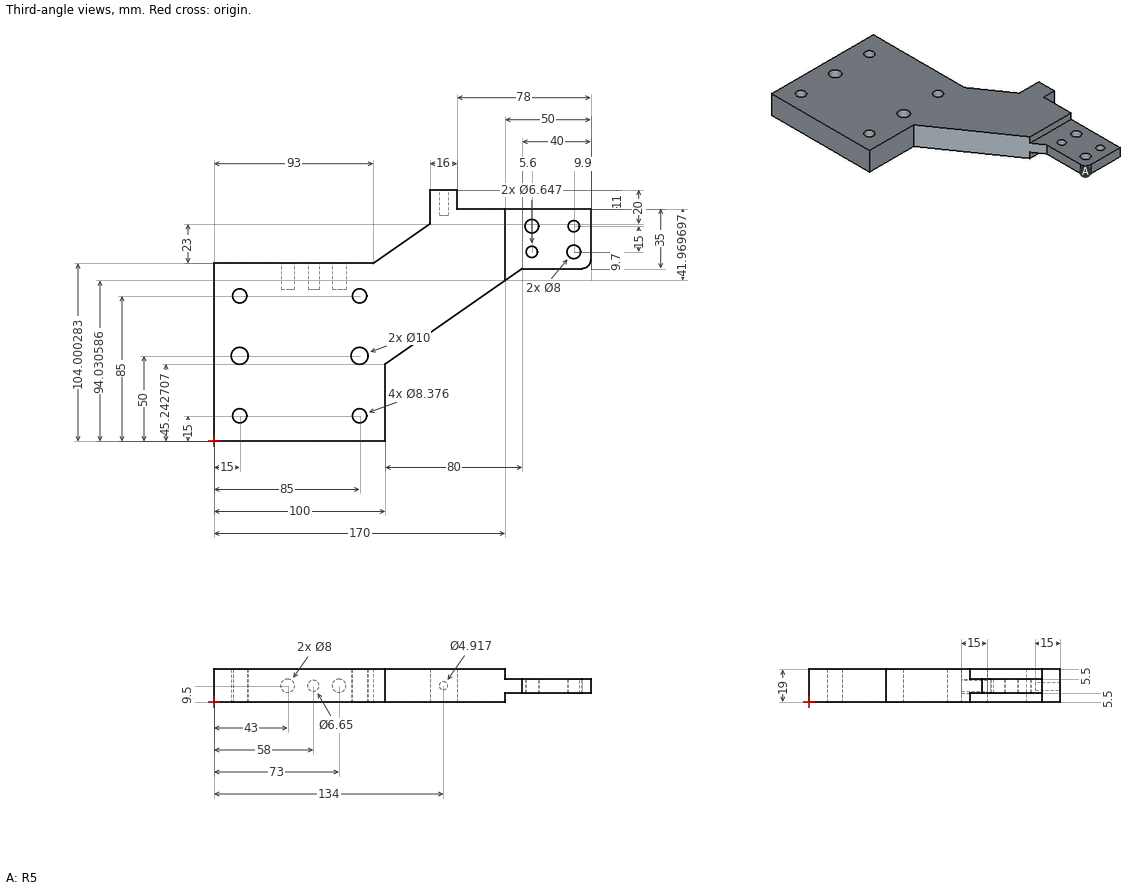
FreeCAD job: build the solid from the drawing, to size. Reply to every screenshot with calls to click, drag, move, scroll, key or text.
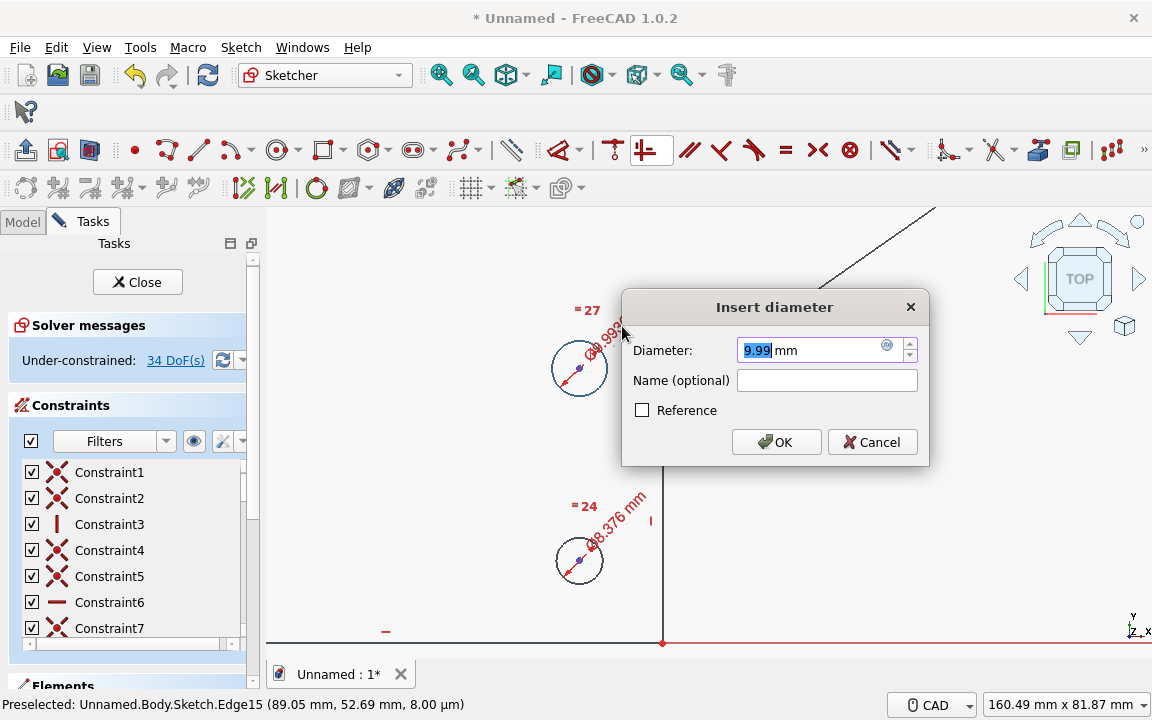
text(10)
key(Return)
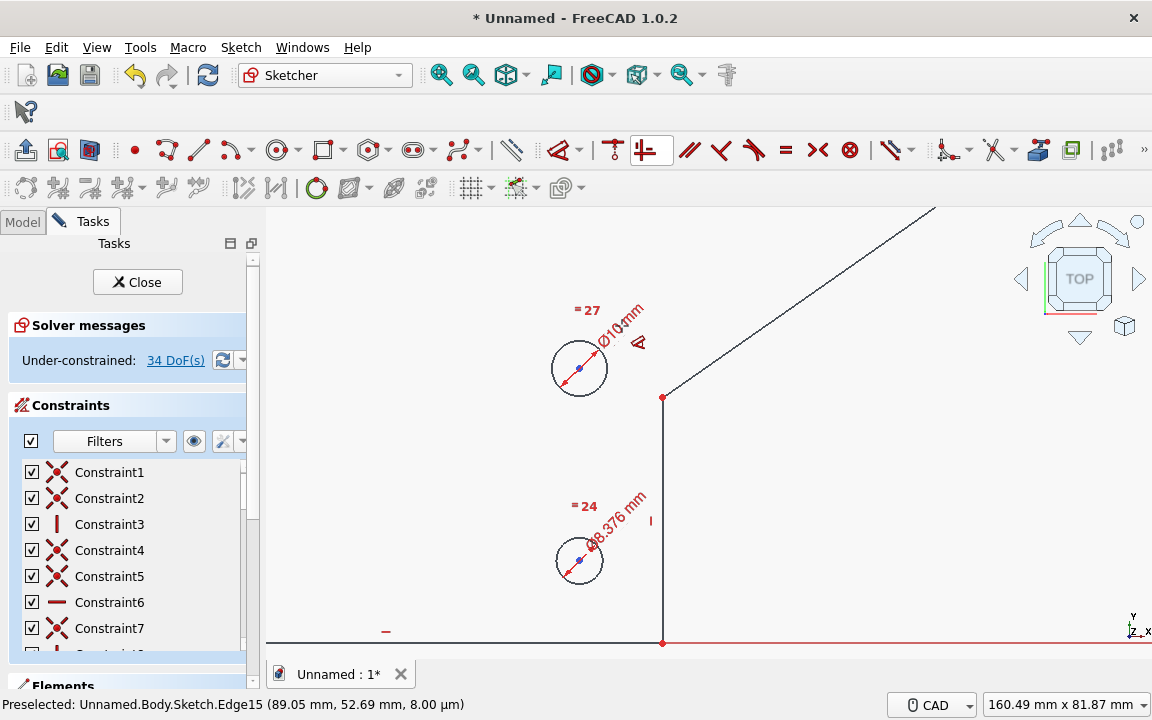
scroll(596, 547, down, 5)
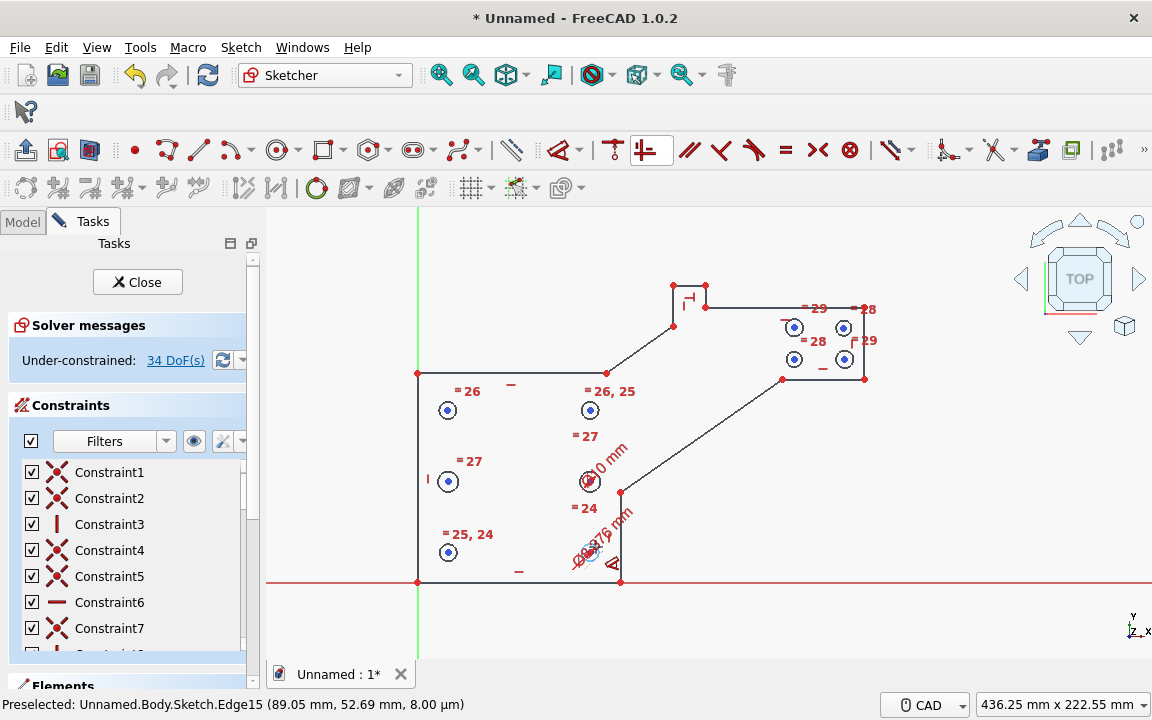
scroll(851, 353, up, 5)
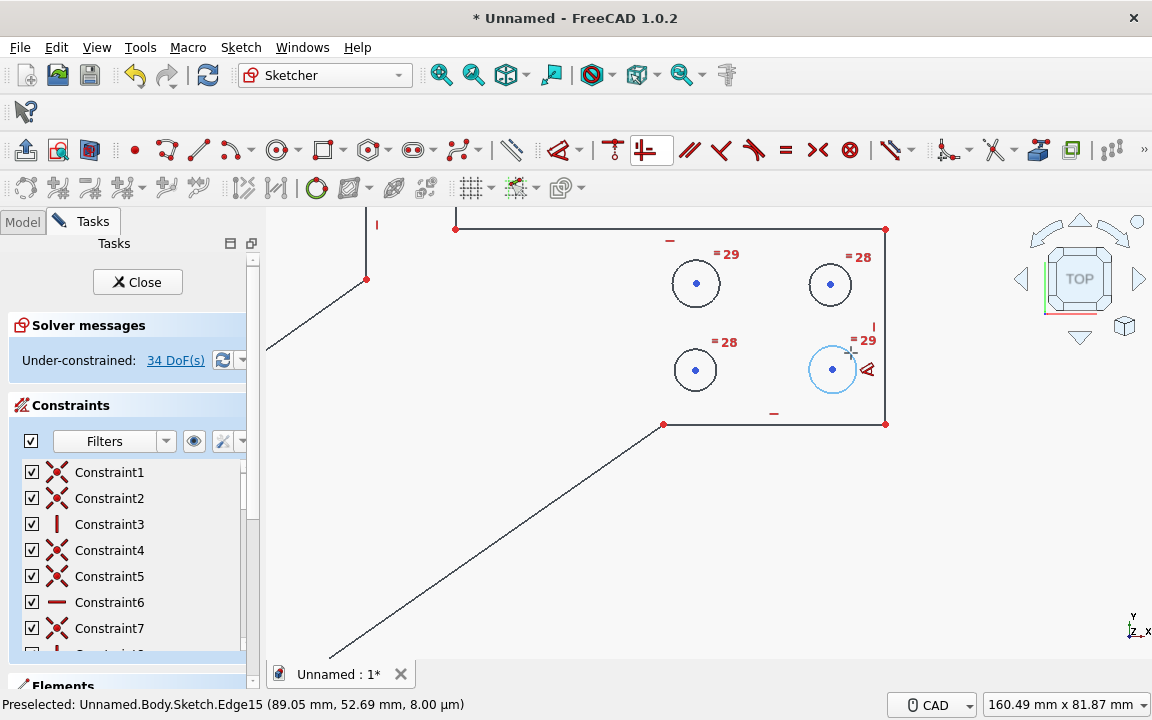
click(849, 353)
click(871, 330)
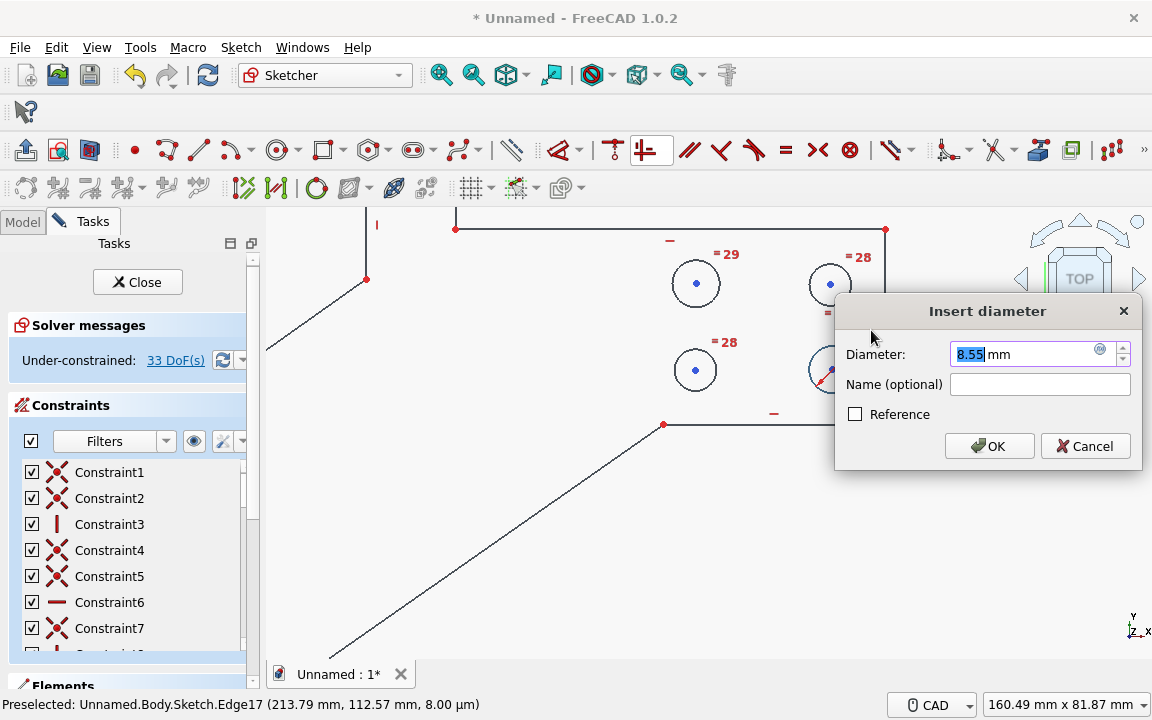
text(8)
key(Return)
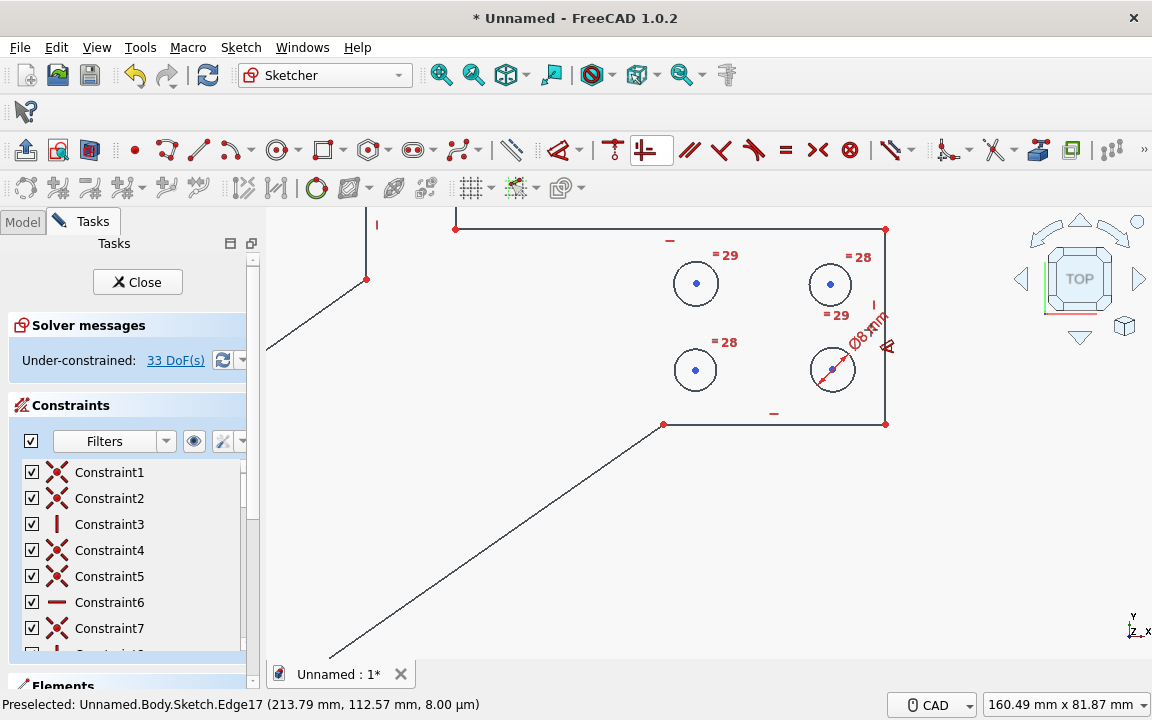
click(710, 355)
click(732, 332)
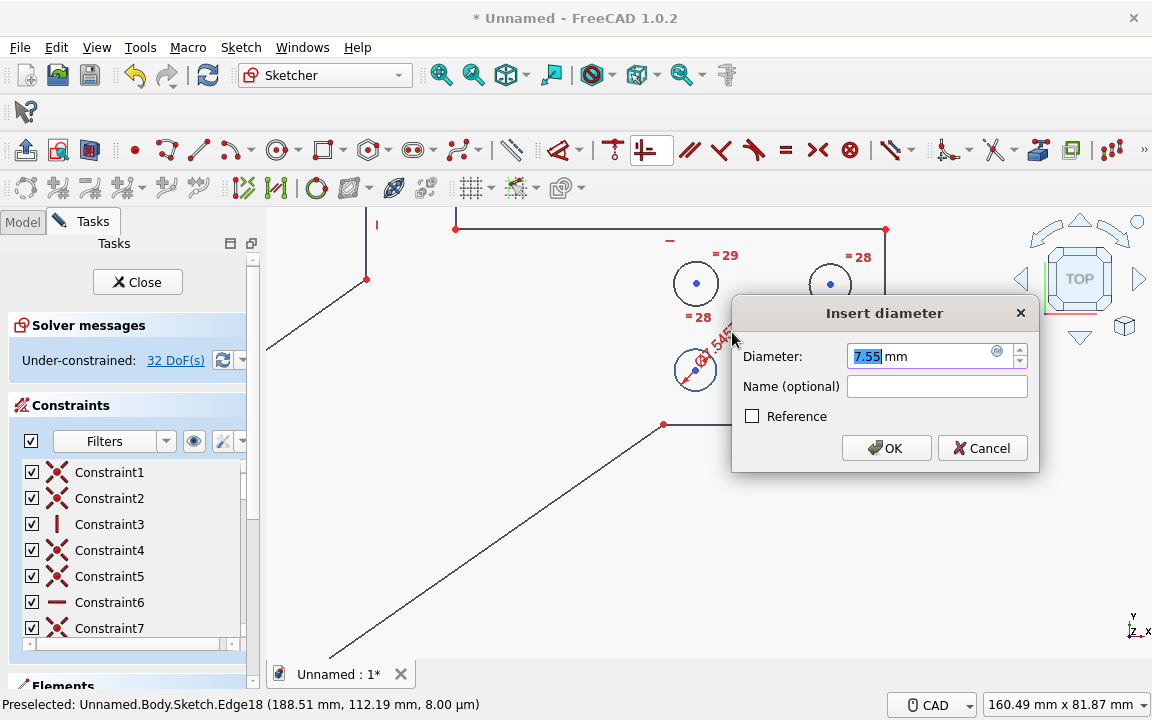
text(6.647)
key(Return)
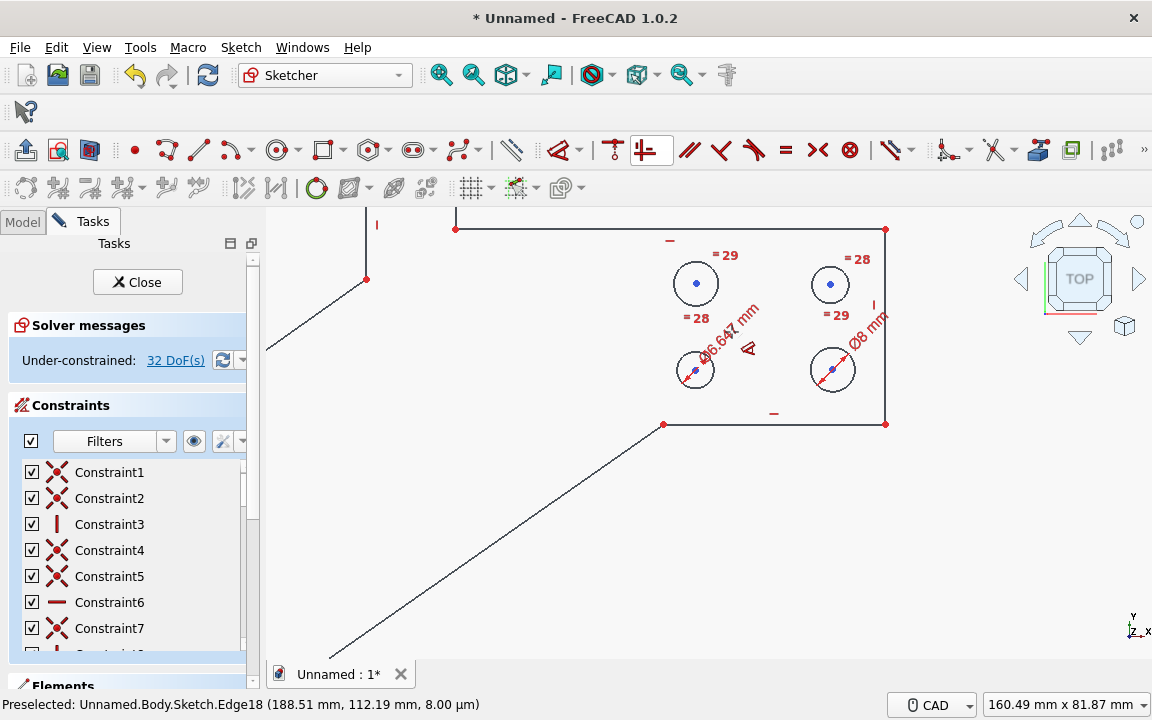
click(730, 425)
click(775, 391)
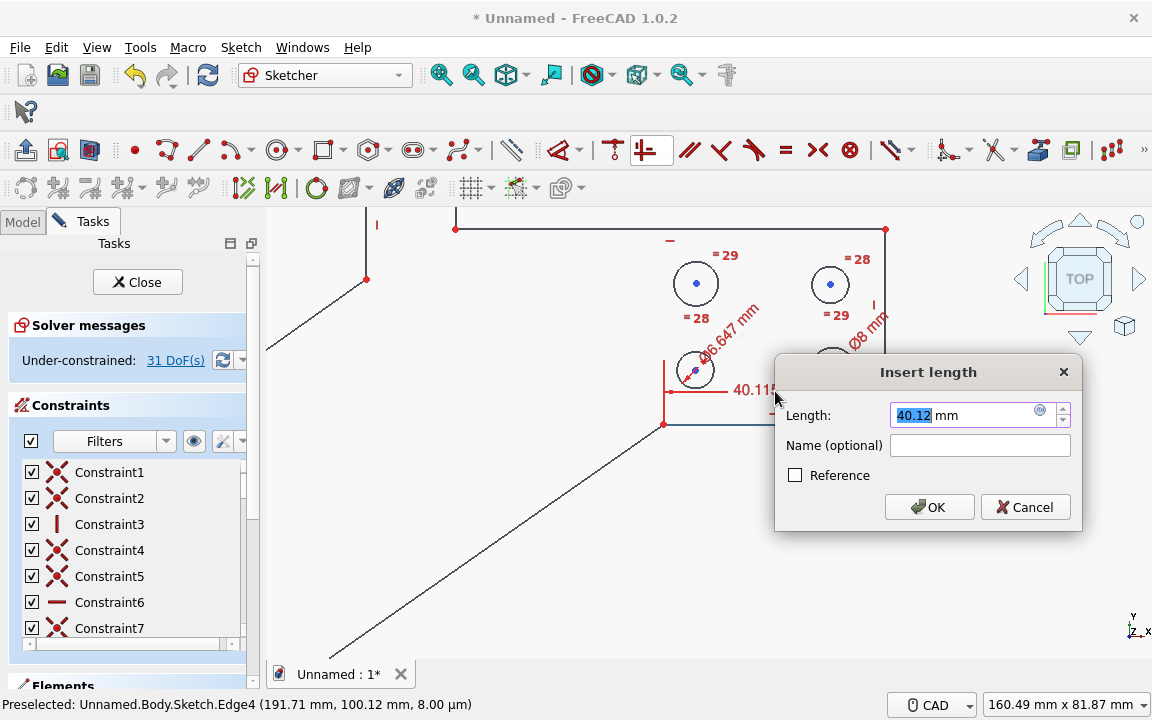
text(40)
key(Return)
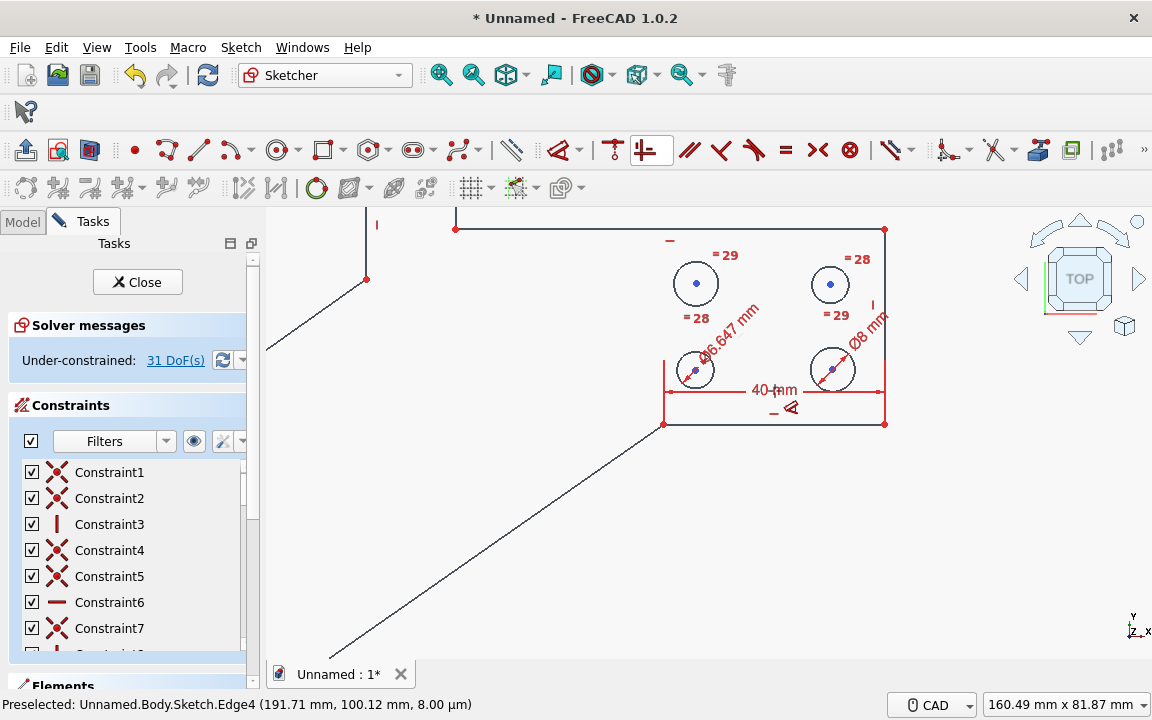
click(885, 366)
click(919, 286)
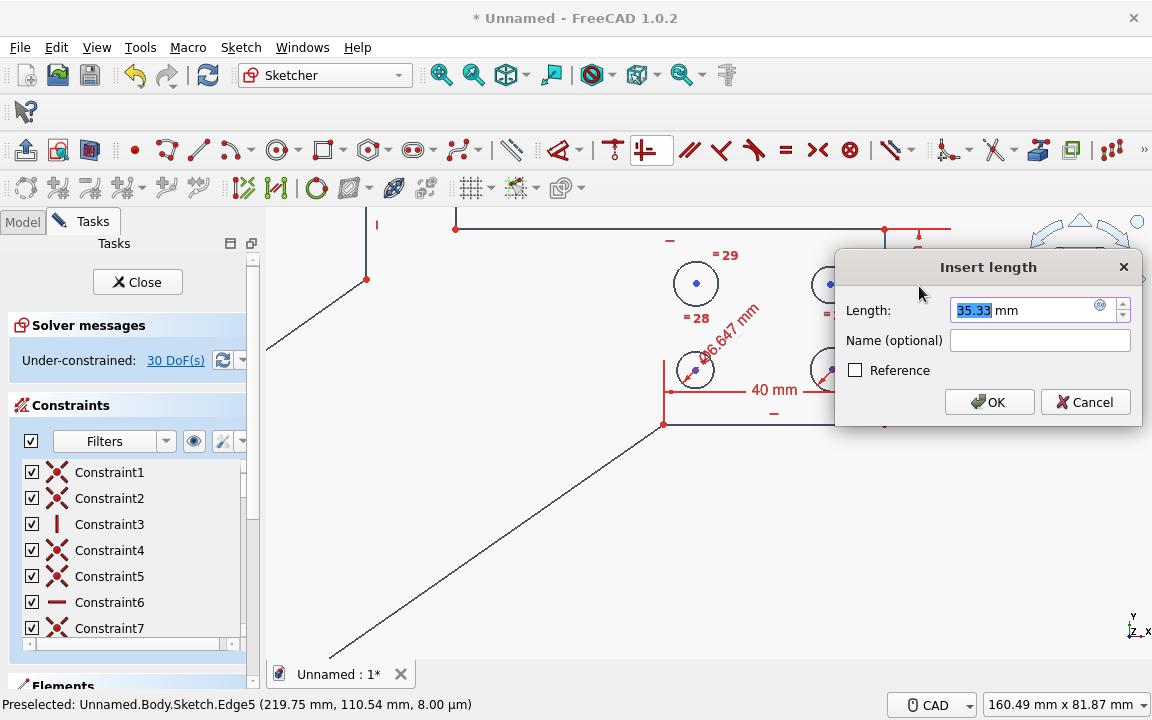
text(35)
key(Return)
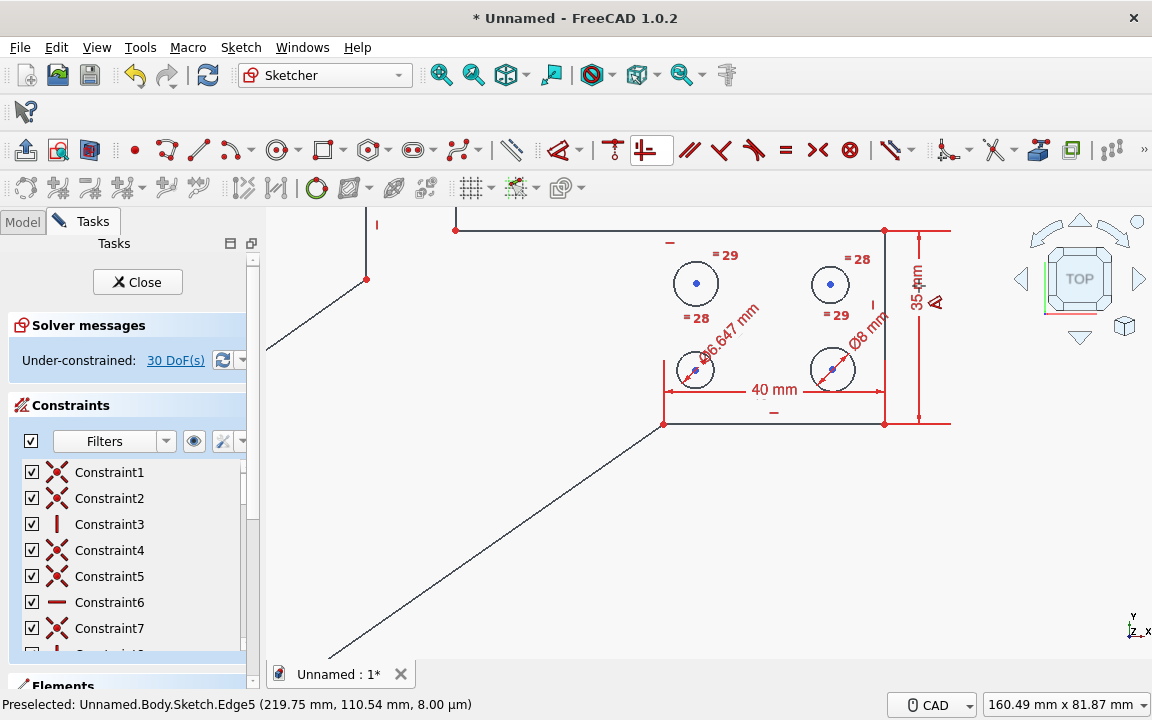
scroll(851, 352, down, 5)